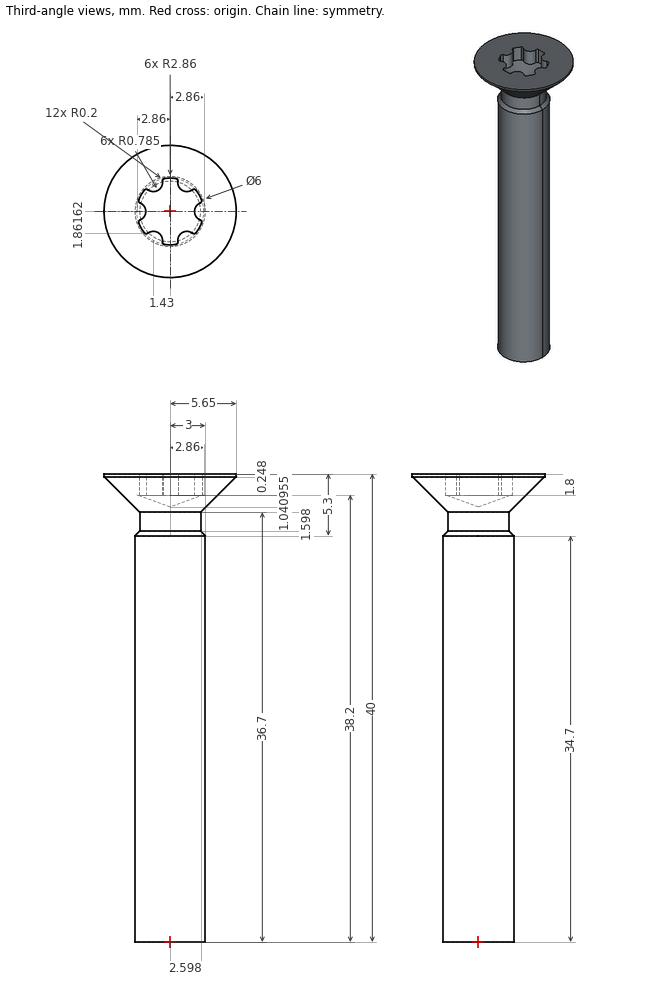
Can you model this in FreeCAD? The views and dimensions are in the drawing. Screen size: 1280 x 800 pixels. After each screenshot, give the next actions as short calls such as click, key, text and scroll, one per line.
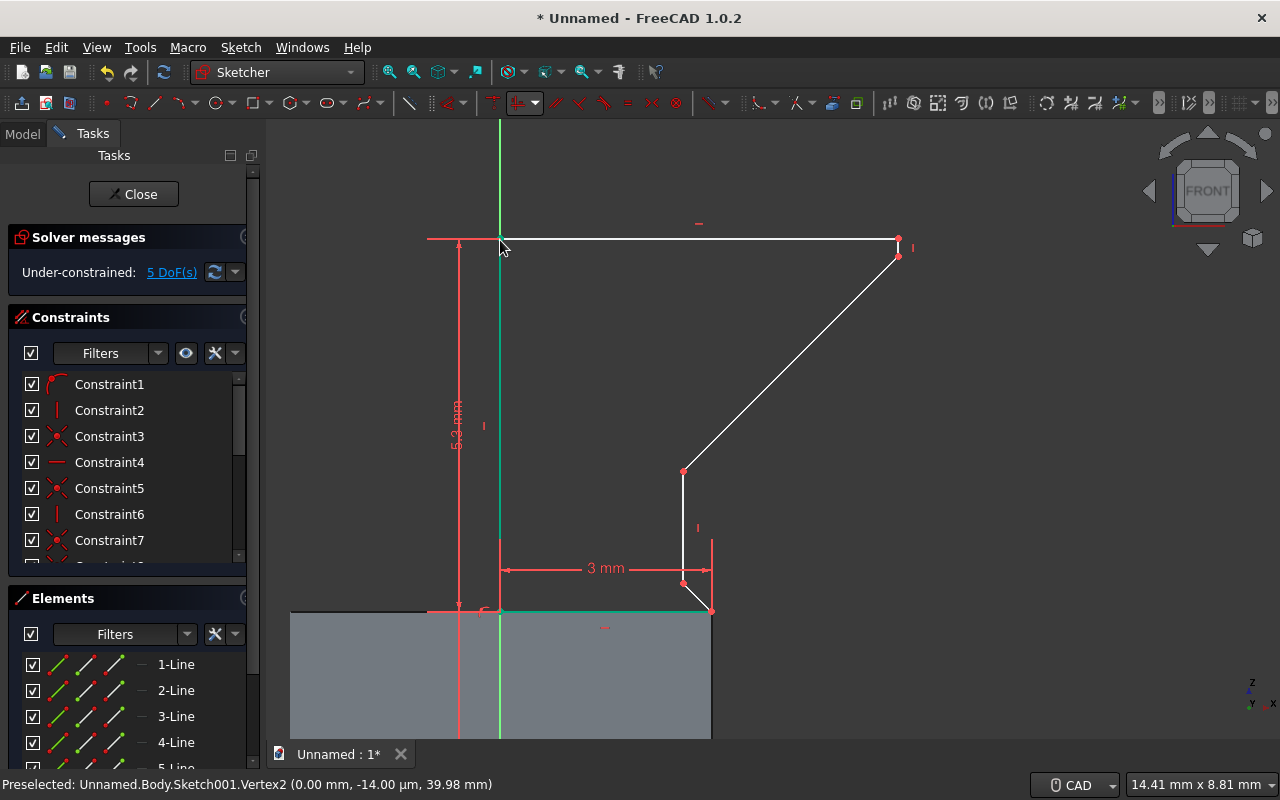
click(620, 239)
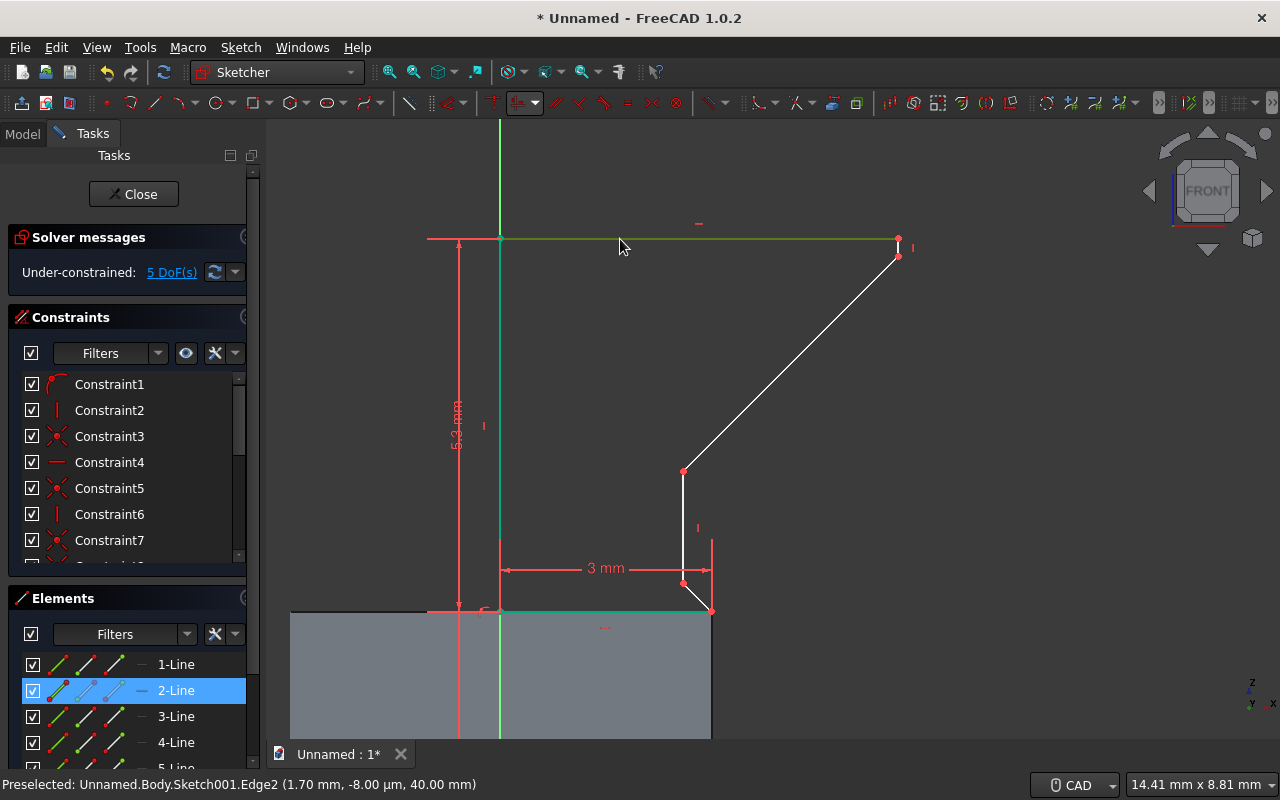
key(l)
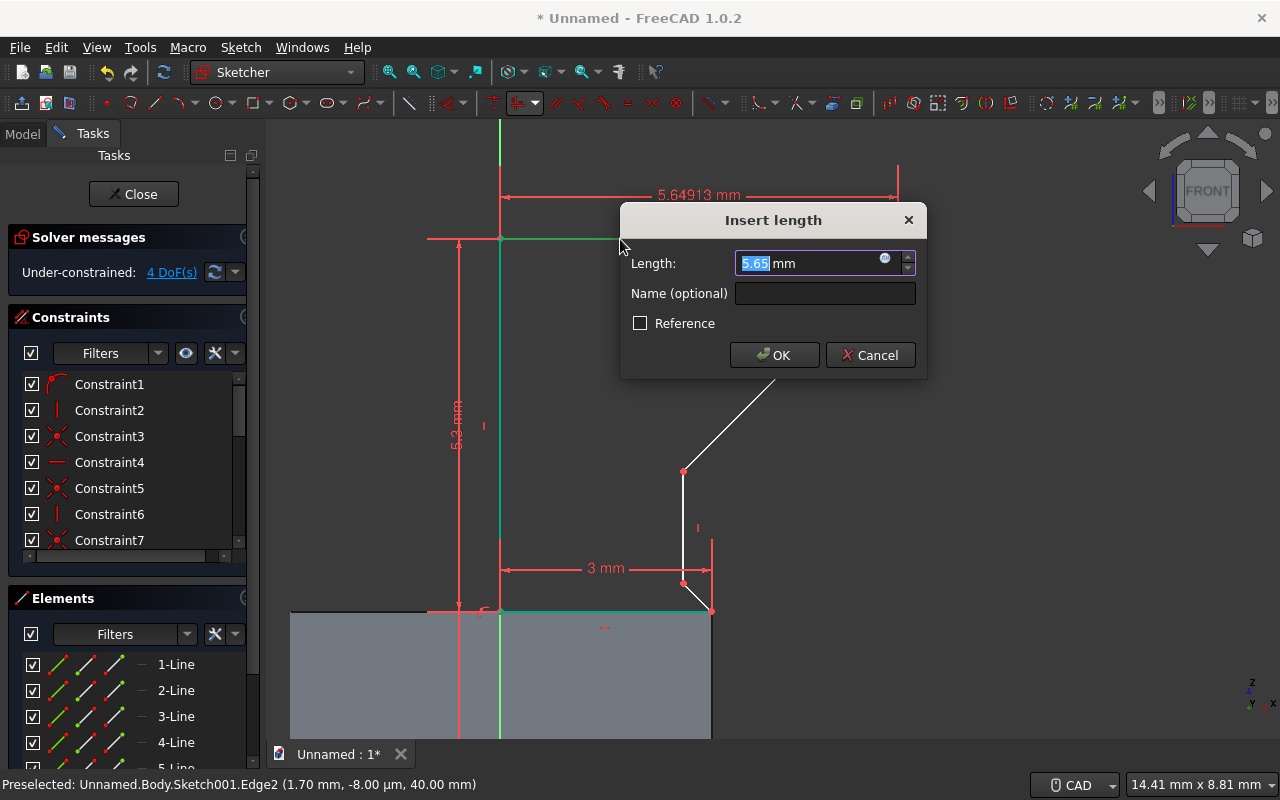
text(5.65)
key(Return)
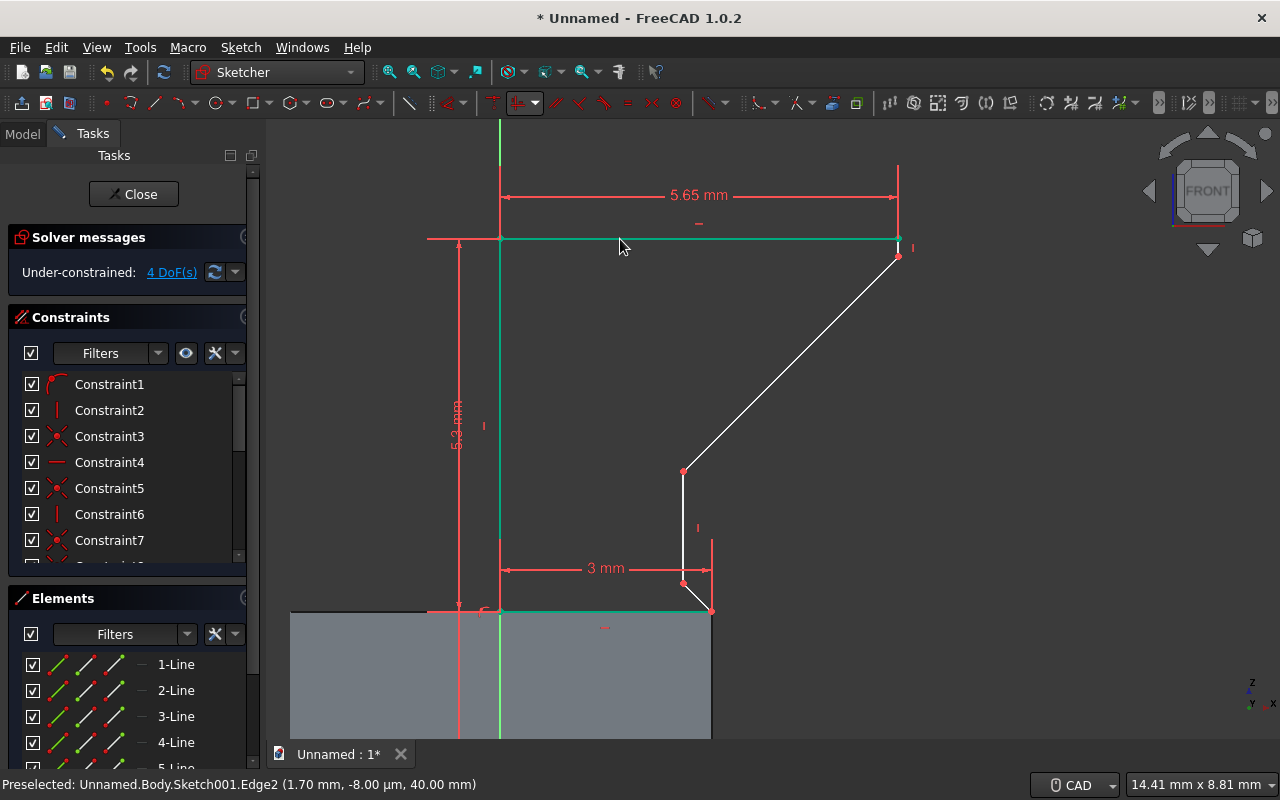
scroll(898, 248, up, 5)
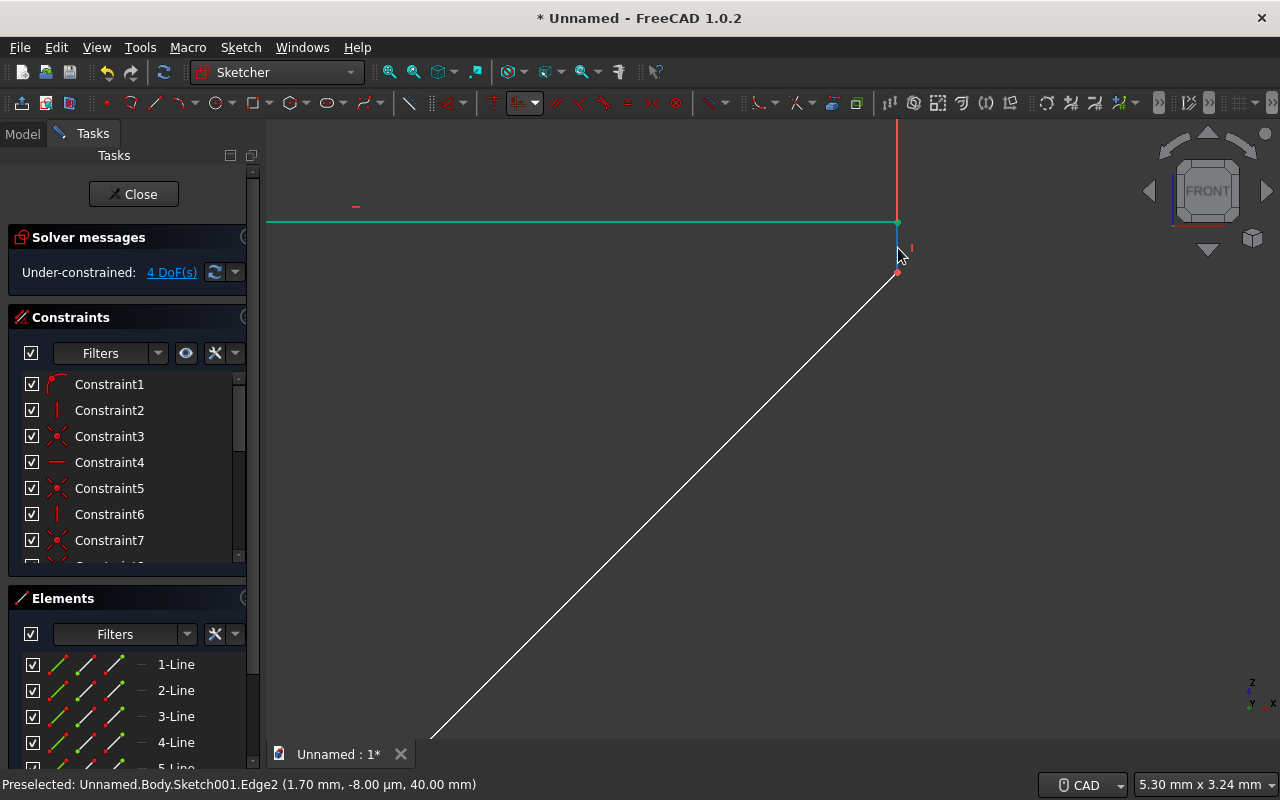
click(897, 247)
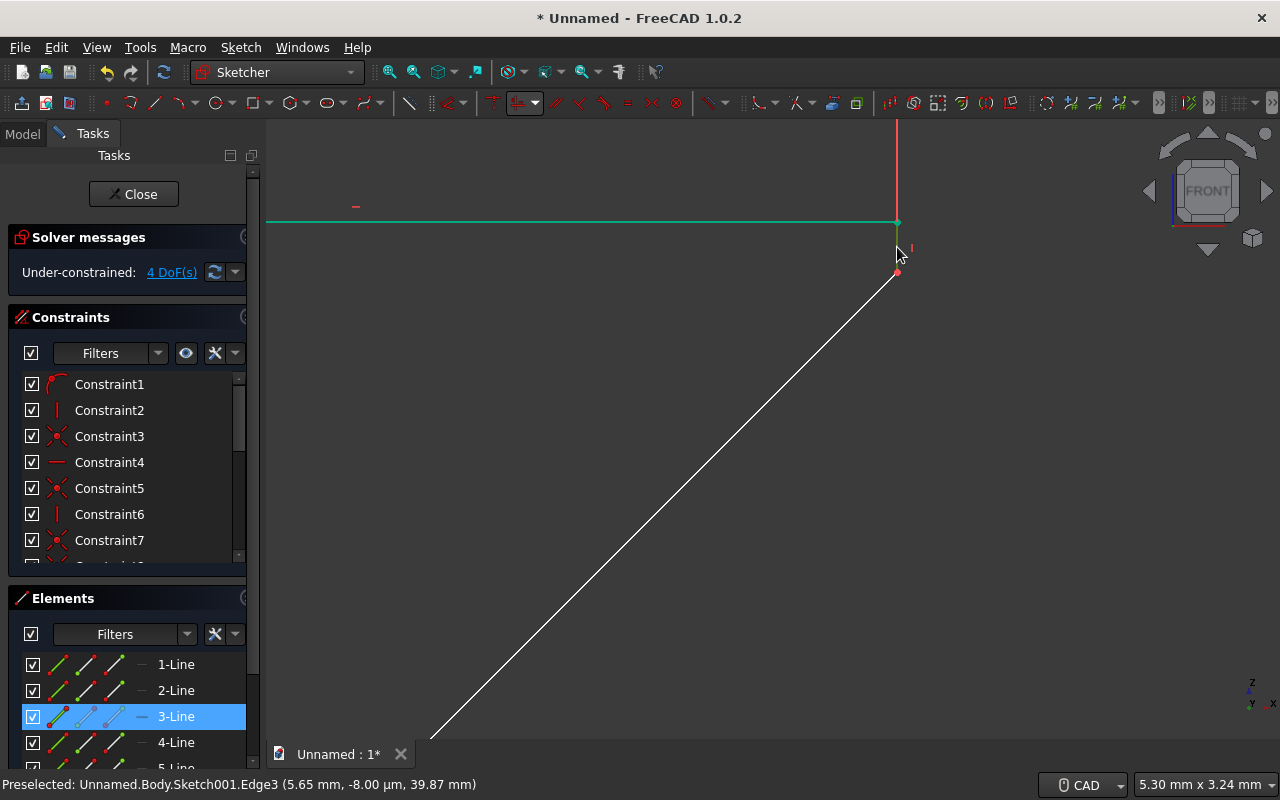
key(i)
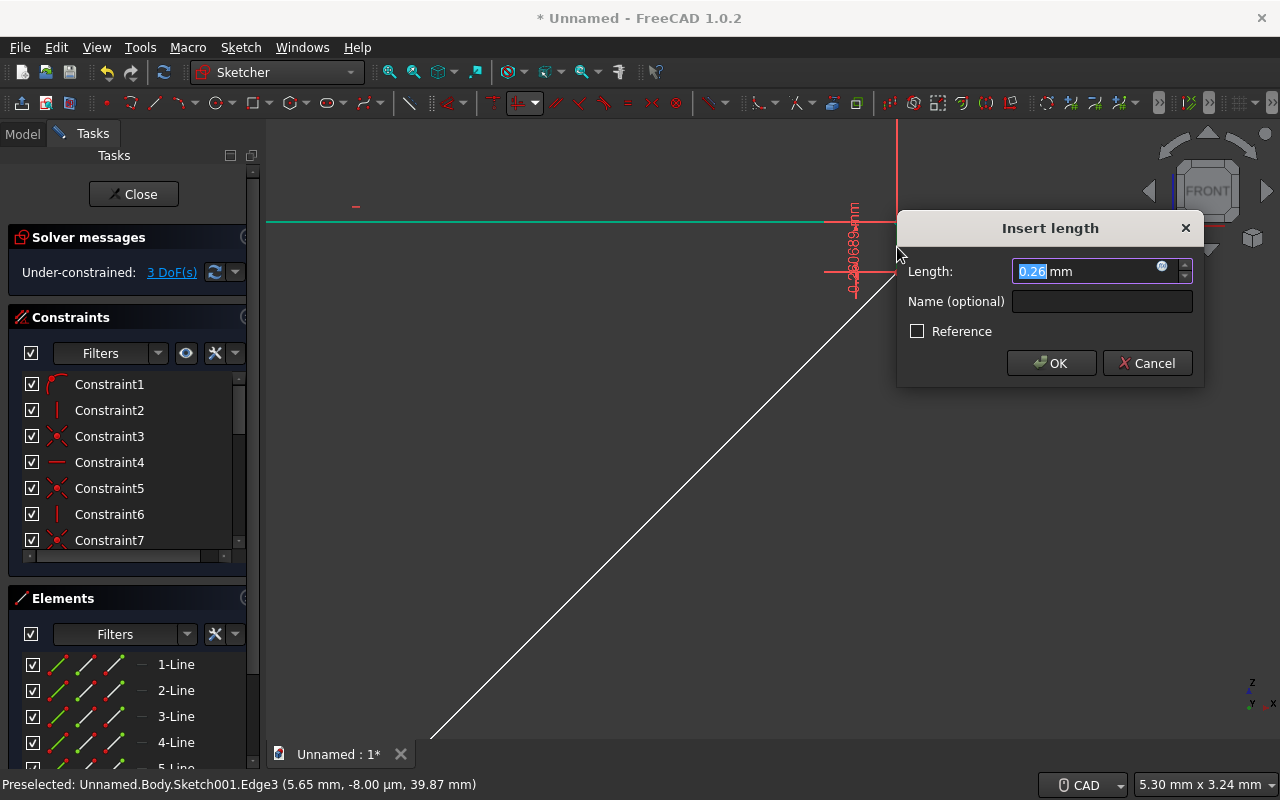
text(0.248)
key(Return)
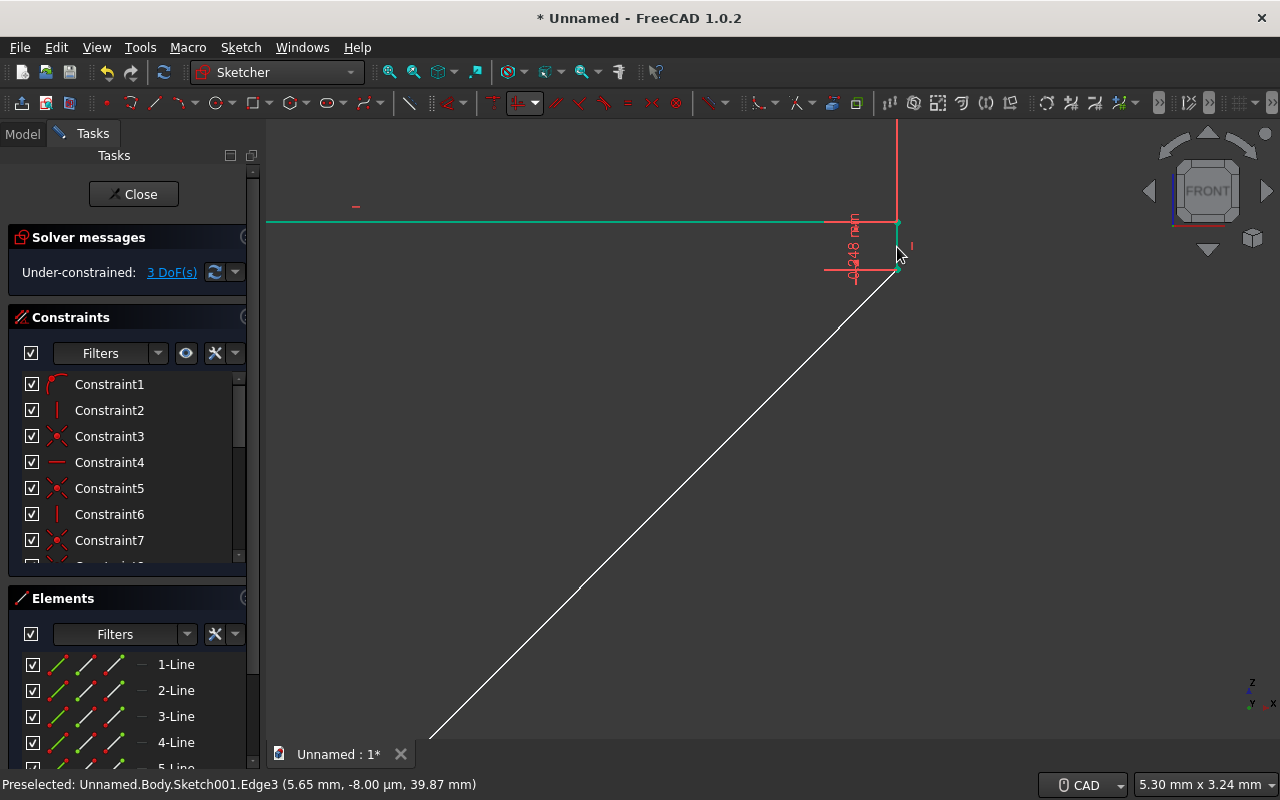
scroll(907, 254, down, 5)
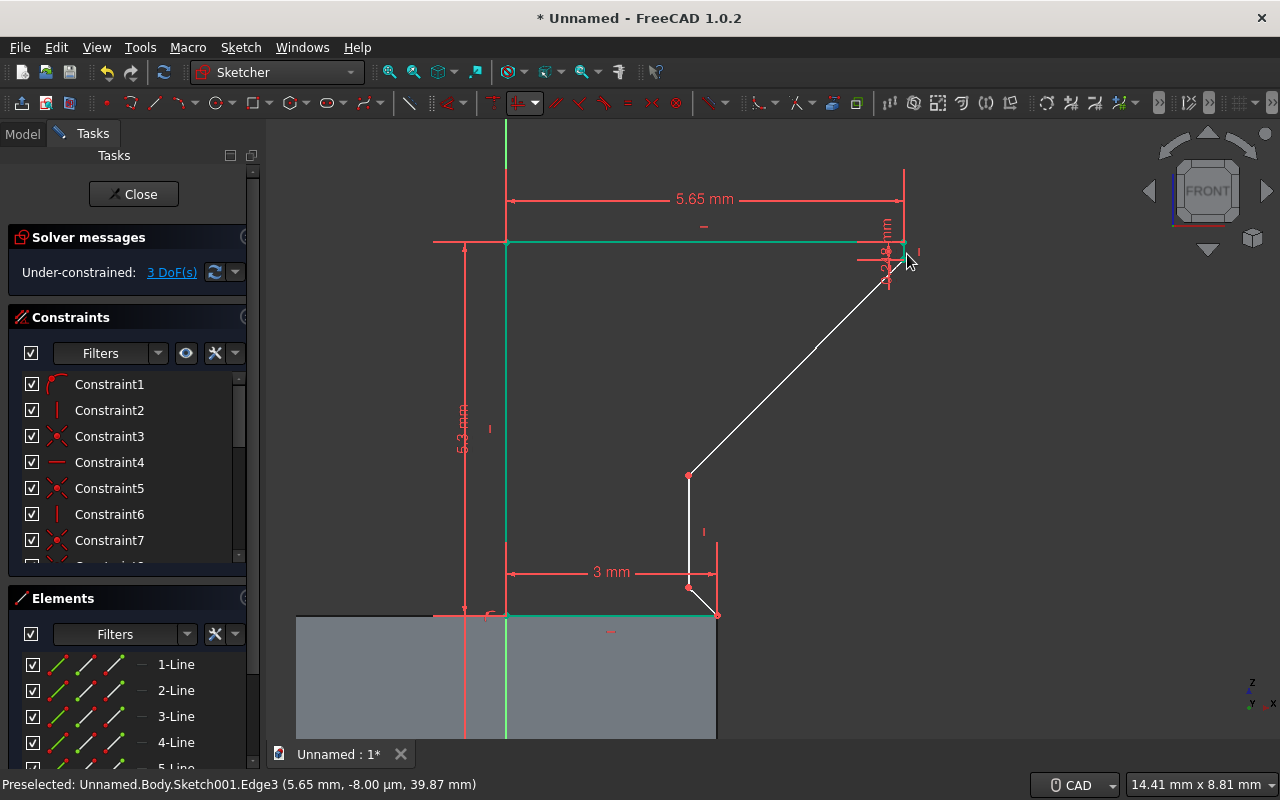
click(689, 509)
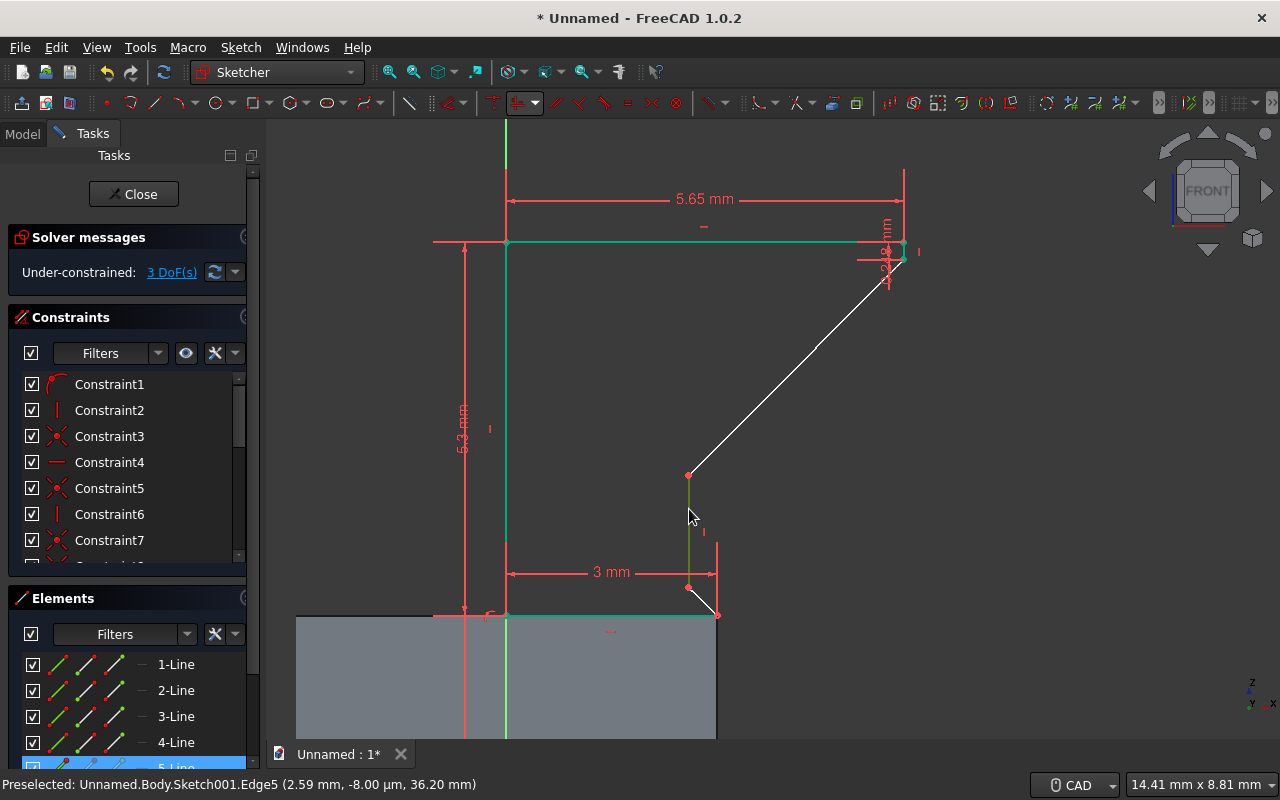
key(i)